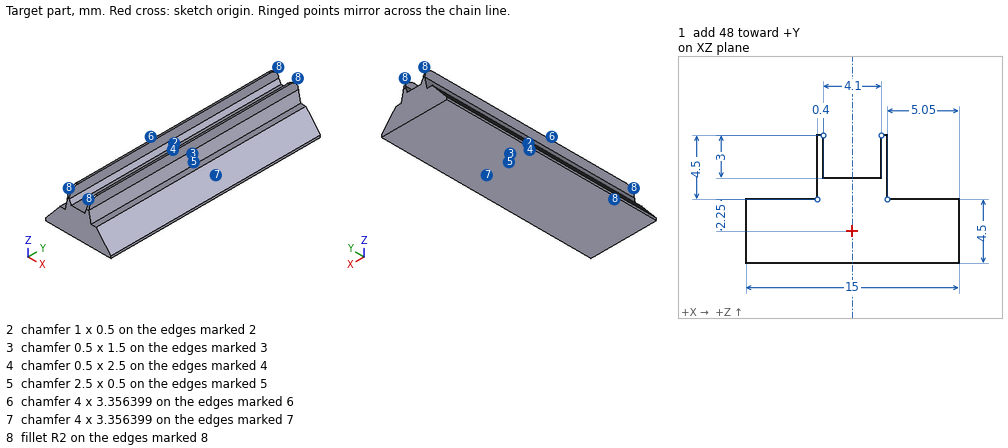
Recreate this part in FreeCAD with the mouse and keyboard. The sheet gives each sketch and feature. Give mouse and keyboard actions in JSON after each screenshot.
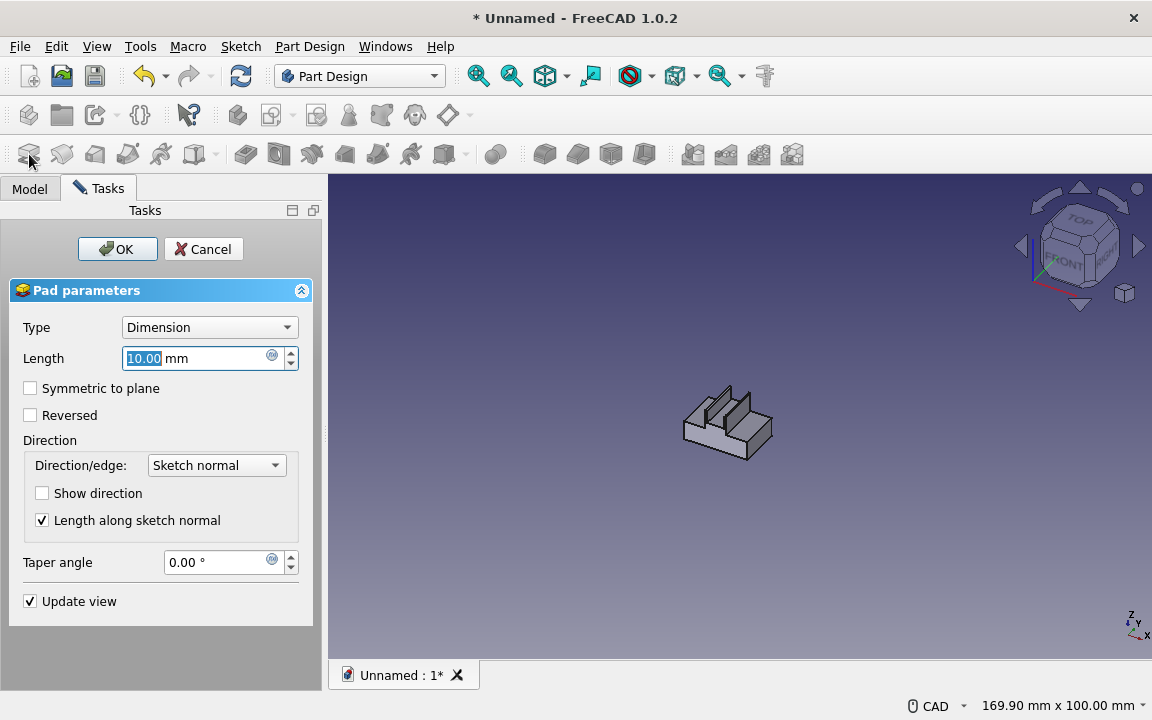
{"action": "type", "text": "48"}
{"action": "key", "text": "Tab"}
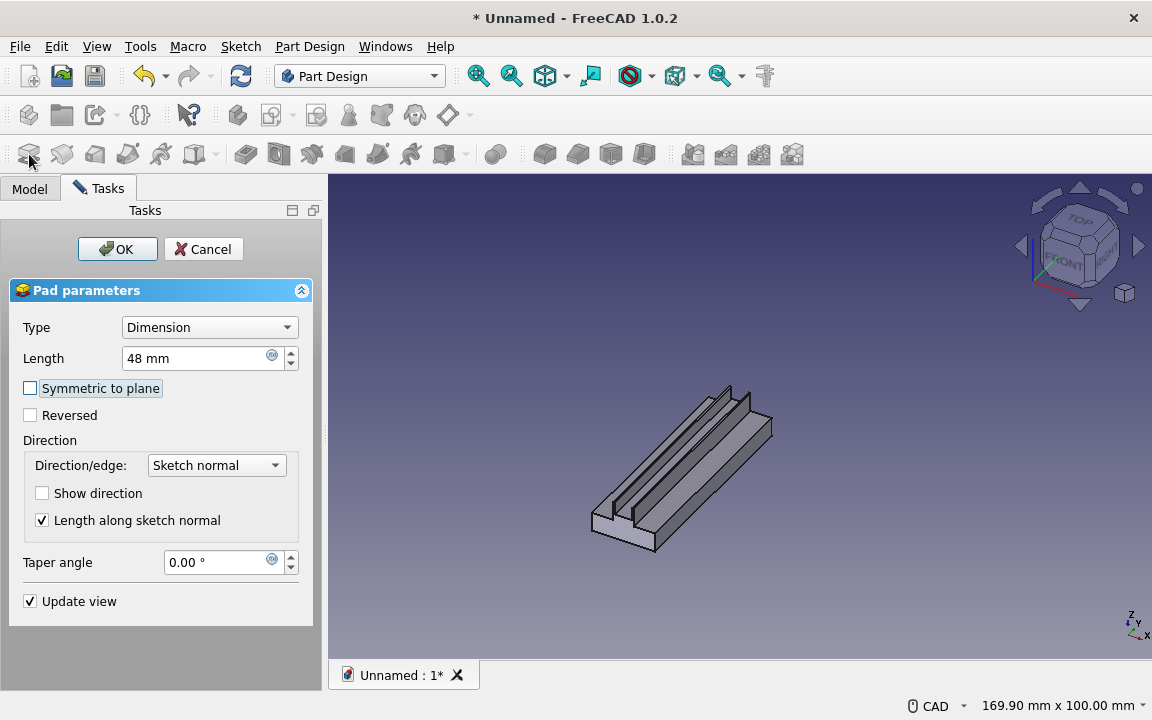
{"action": "left_click", "coordinate": [31, 415]}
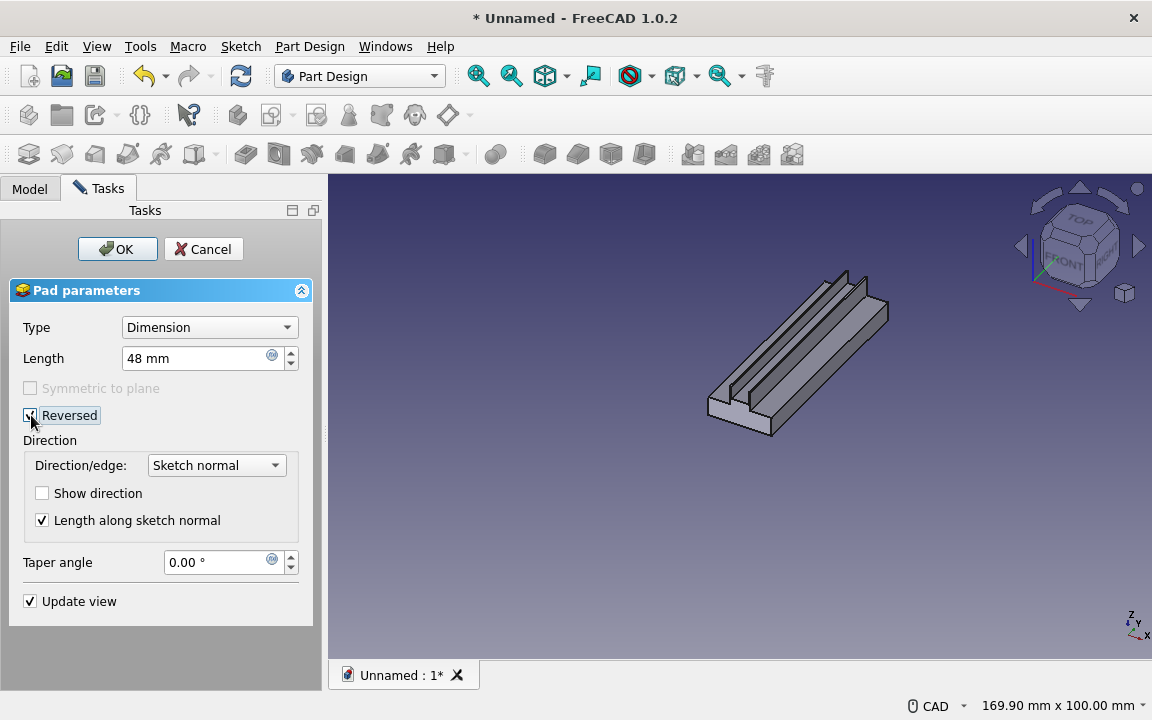
{"action": "left_click", "coordinate": [118, 249]}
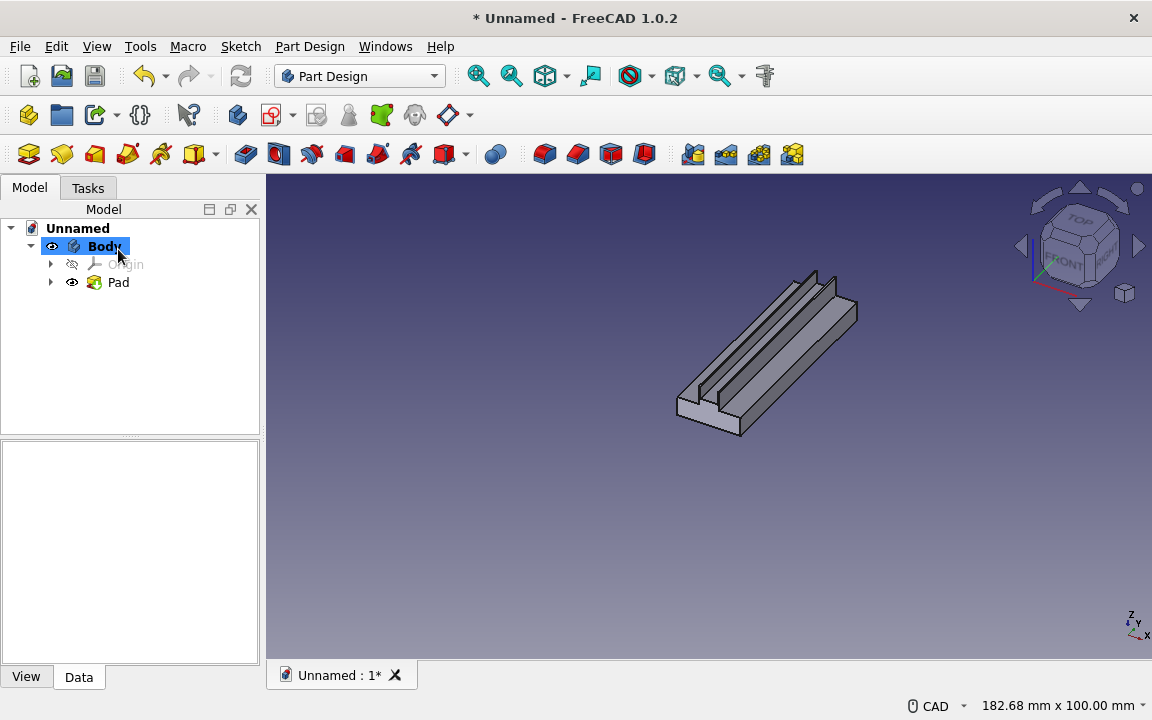
{"action": "left_click", "coordinate": [479, 76]}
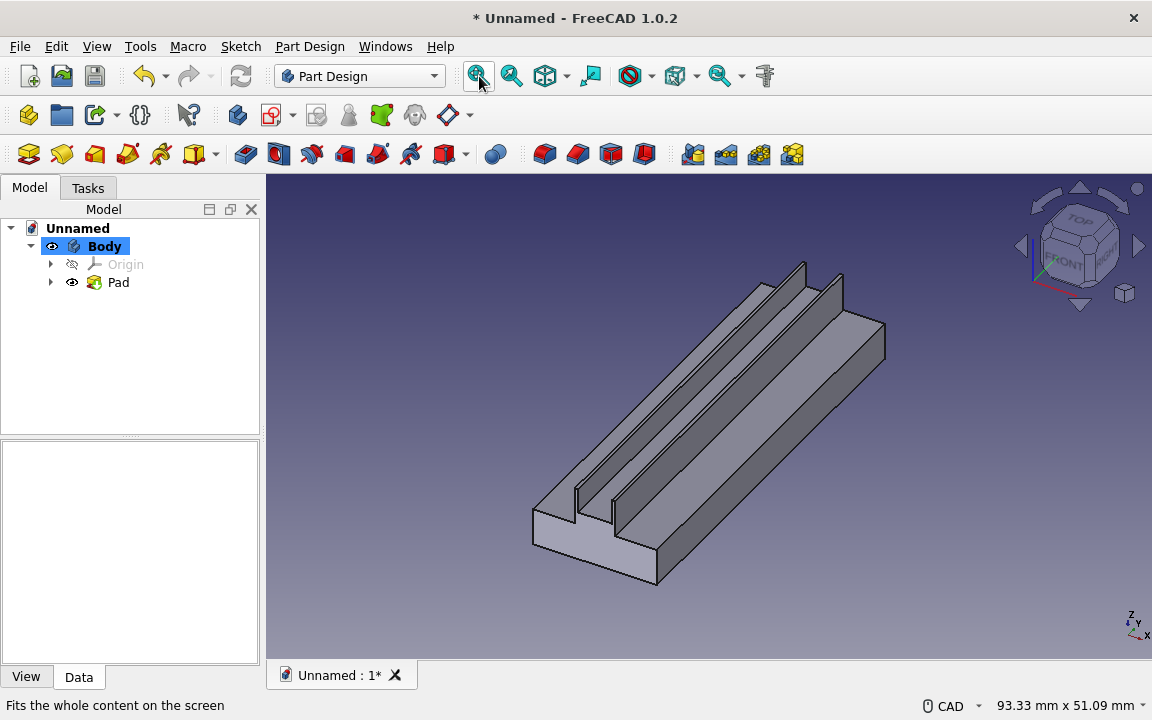
{"action": "key", "text": "0"}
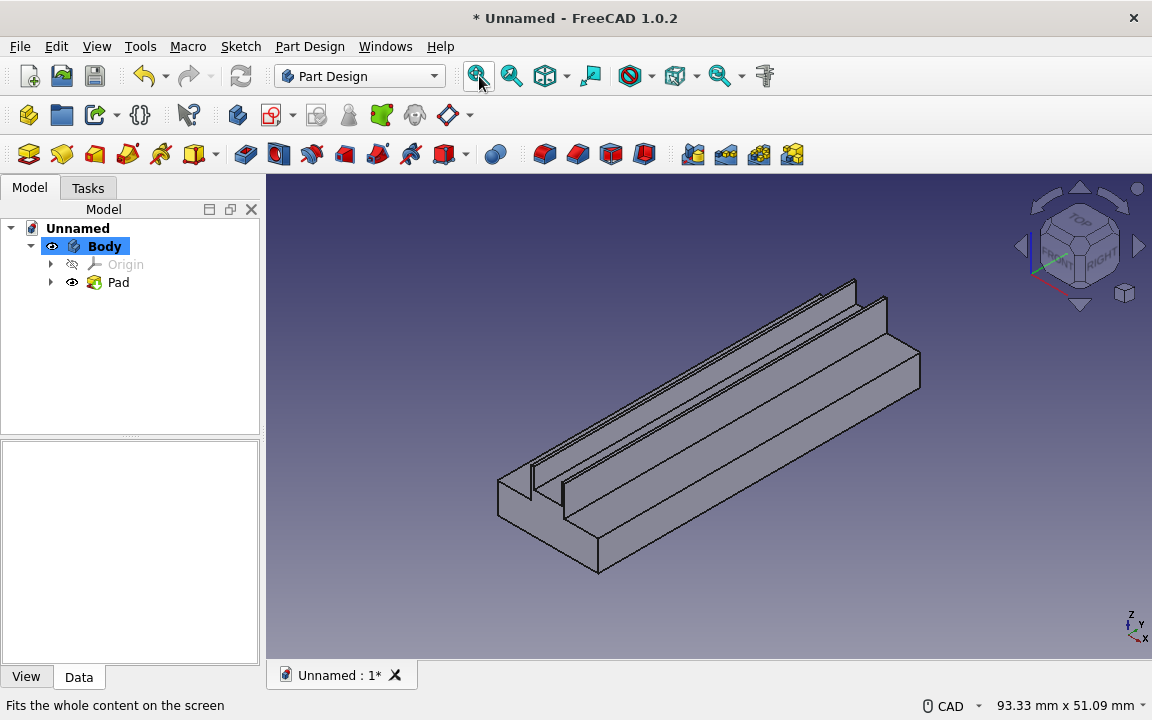
{"action": "key", "text": "2"}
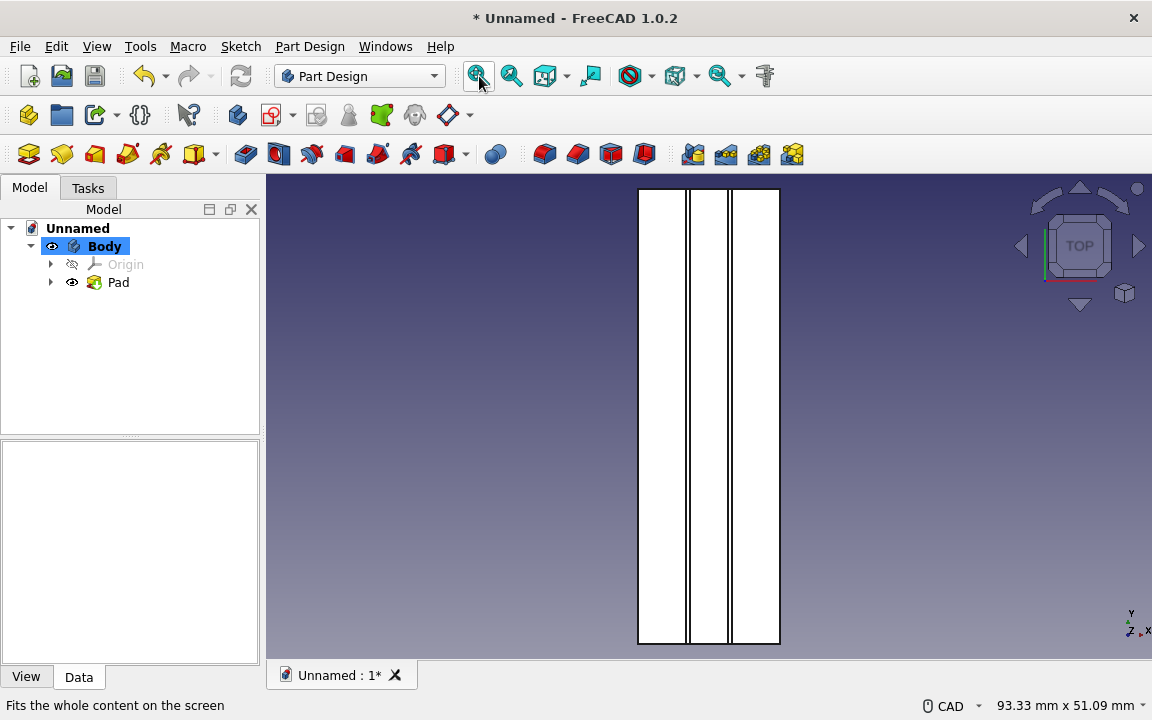
{"action": "key", "text": "1"}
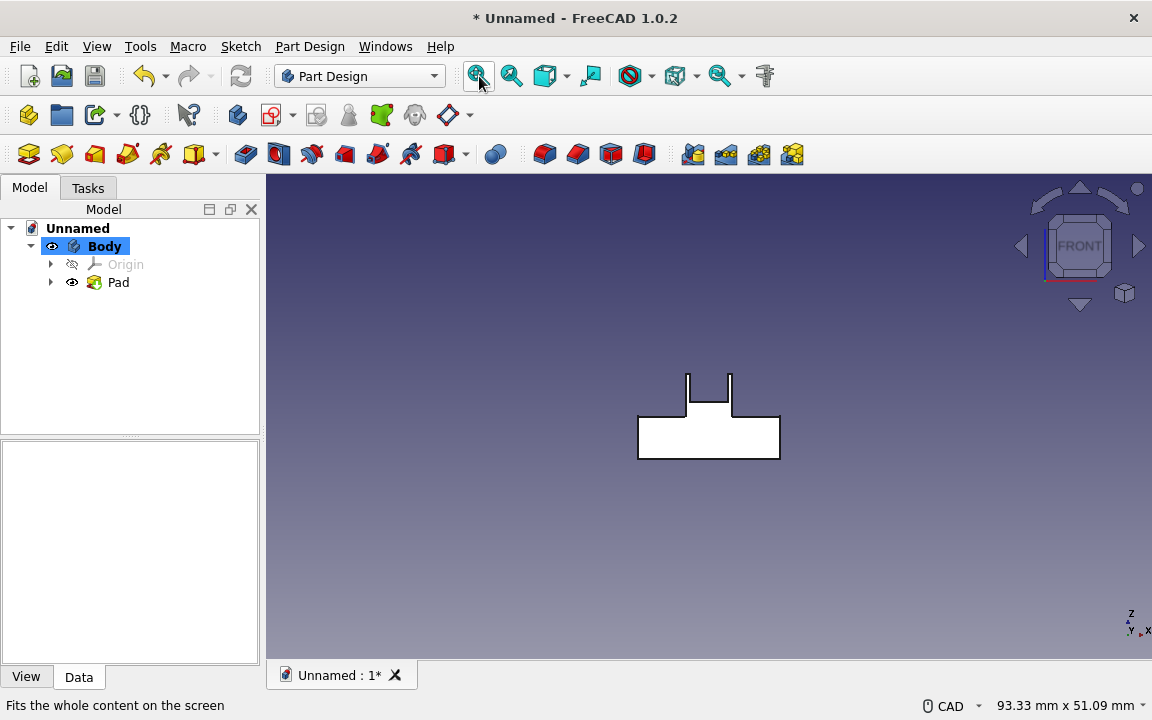
{"action": "left_click", "coordinate": [479, 76]}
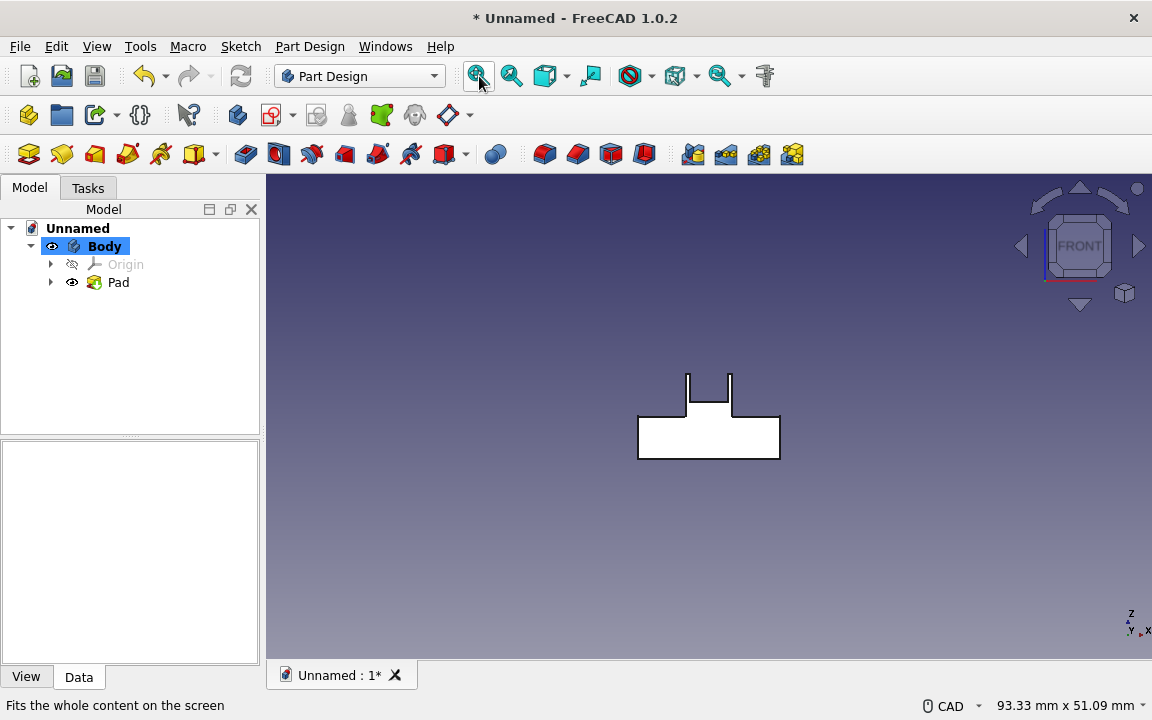
{"action": "key", "text": "3"}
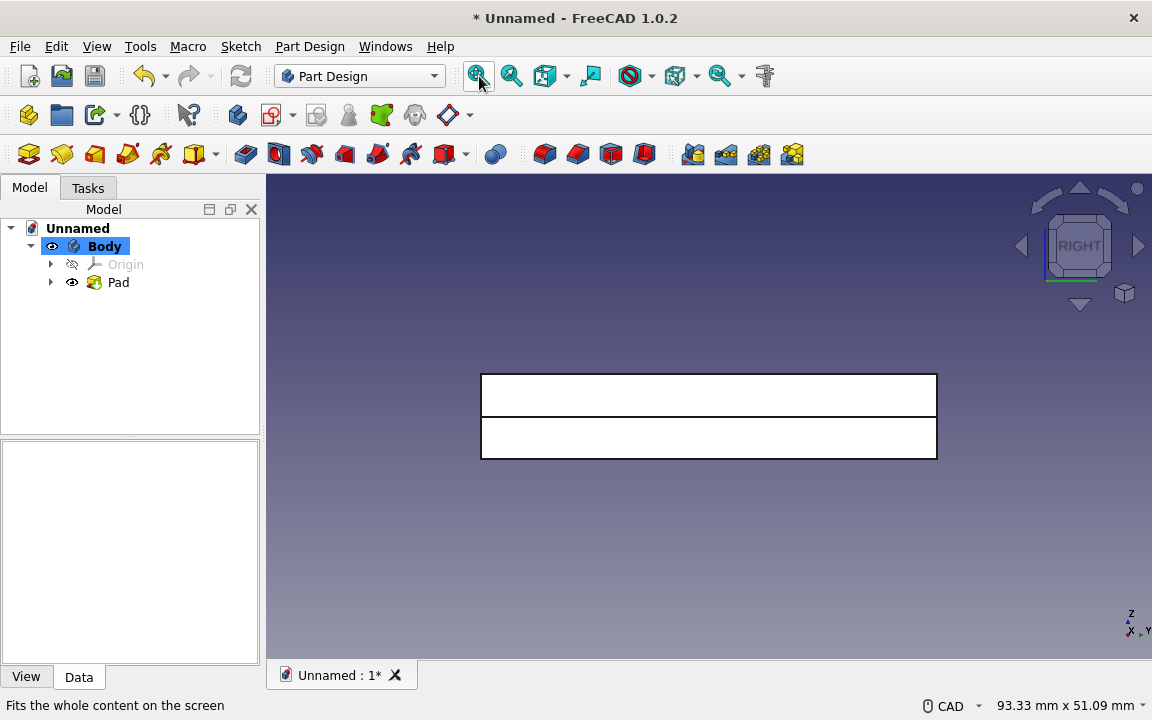
{"action": "key", "text": "5"}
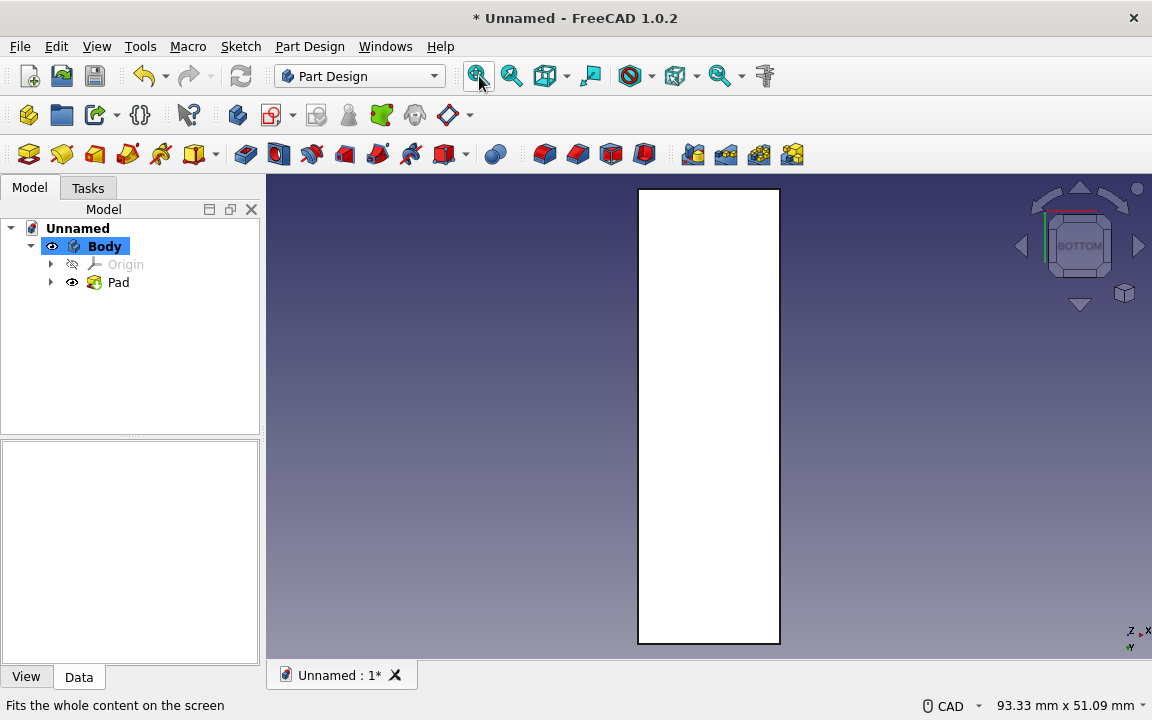
{"action": "key", "text": "4"}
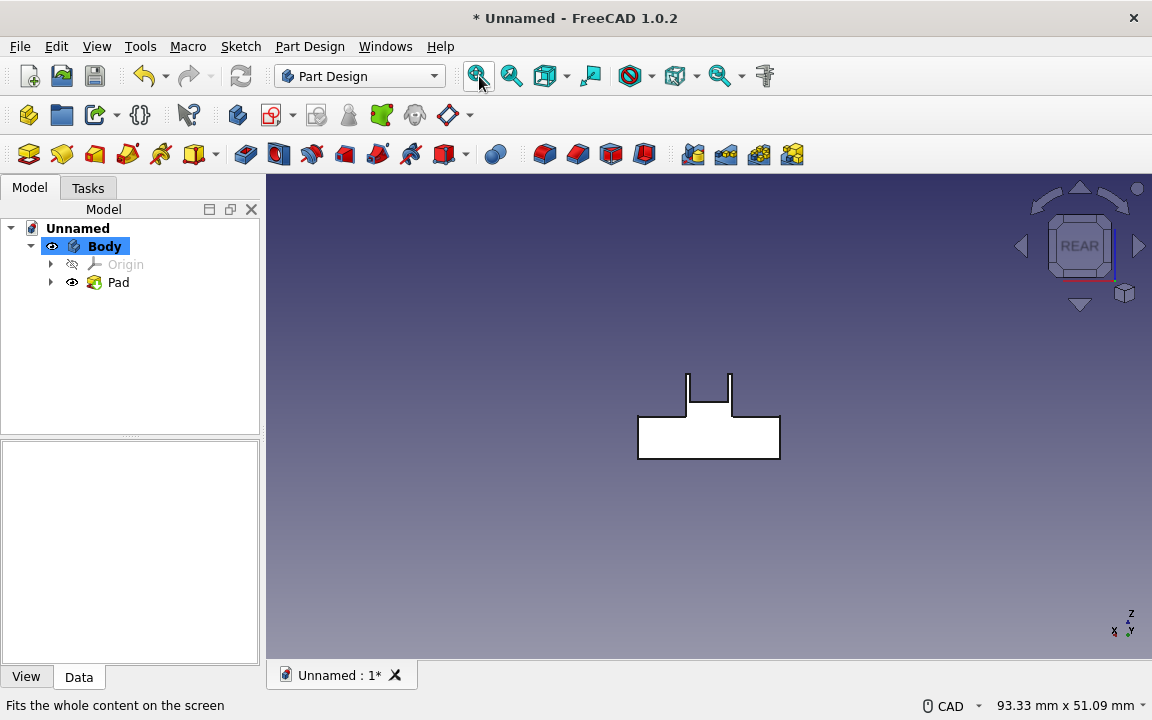
{"action": "left_click", "coordinate": [479, 76]}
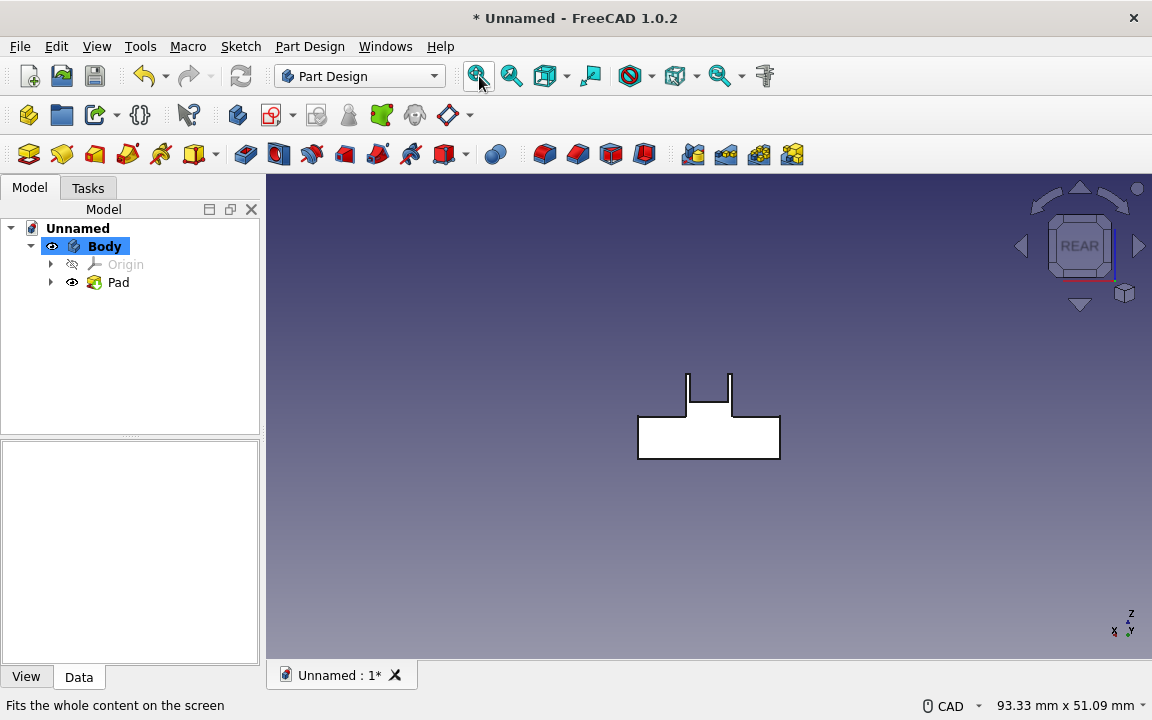
{"action": "key", "text": "6"}